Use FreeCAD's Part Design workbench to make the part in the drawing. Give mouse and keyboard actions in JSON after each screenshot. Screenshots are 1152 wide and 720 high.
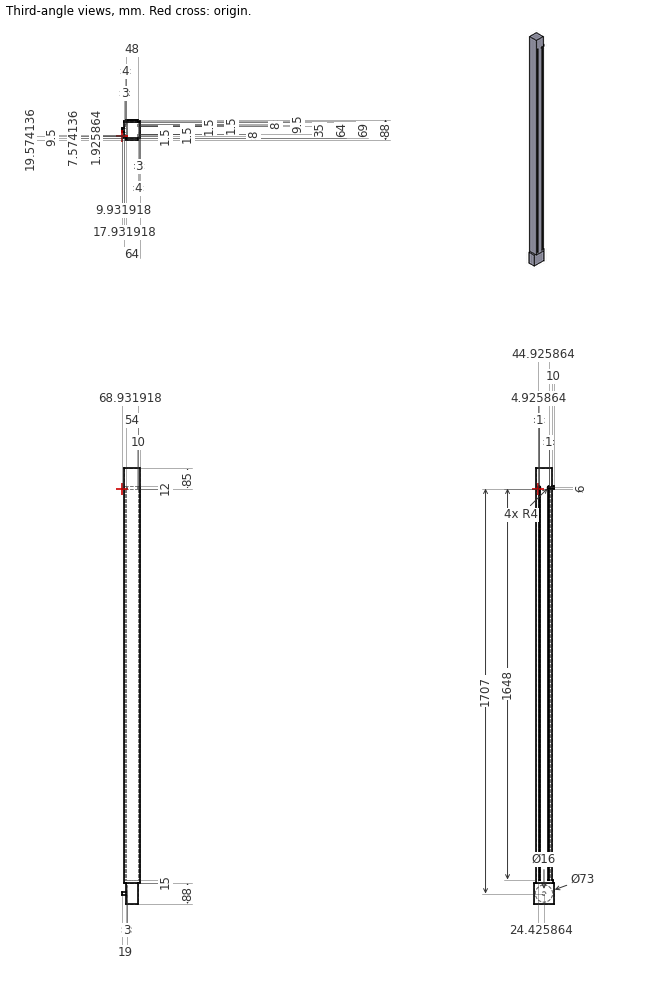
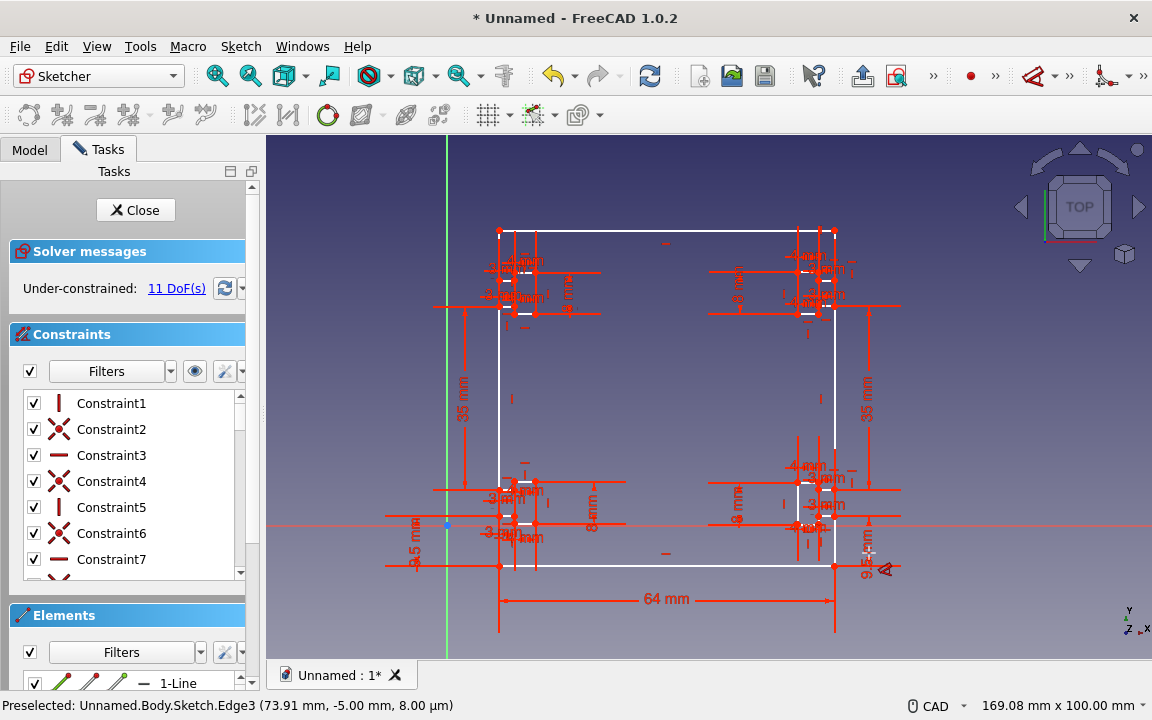
{"action": "scroll", "coordinate": [819, 520], "scroll_direction": "up", "scroll_amount": 9}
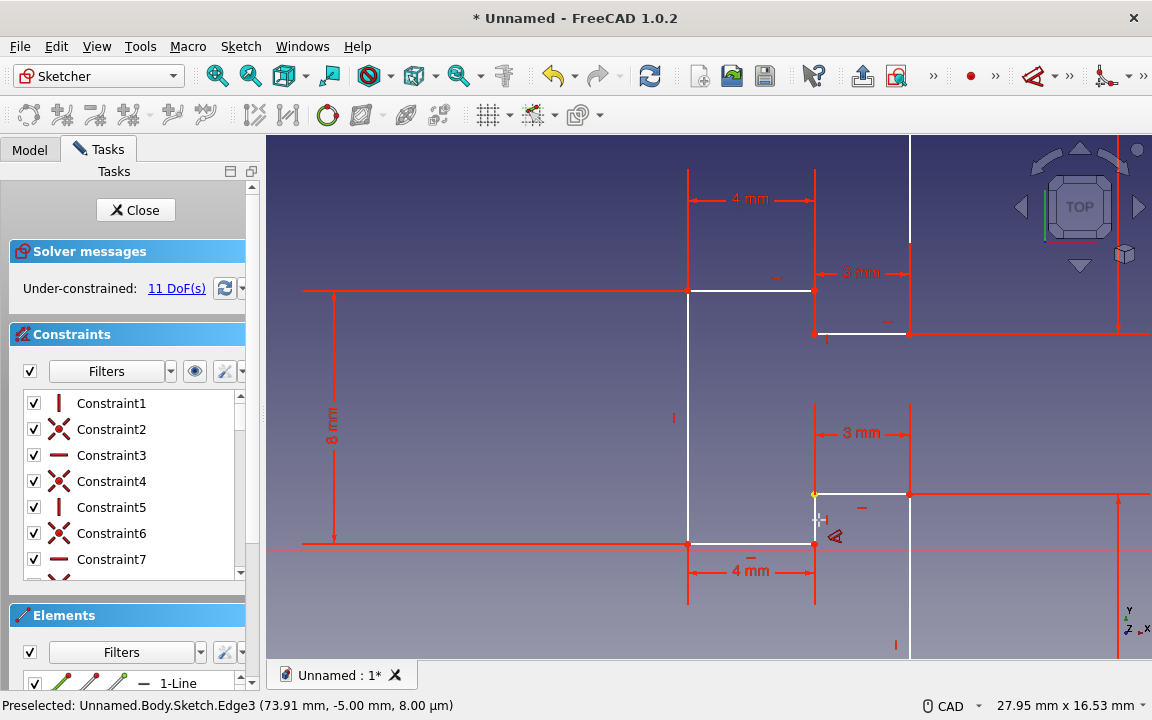
{"action": "left_click", "coordinate": [815, 519]}
{"action": "left_click", "coordinate": [849, 519]}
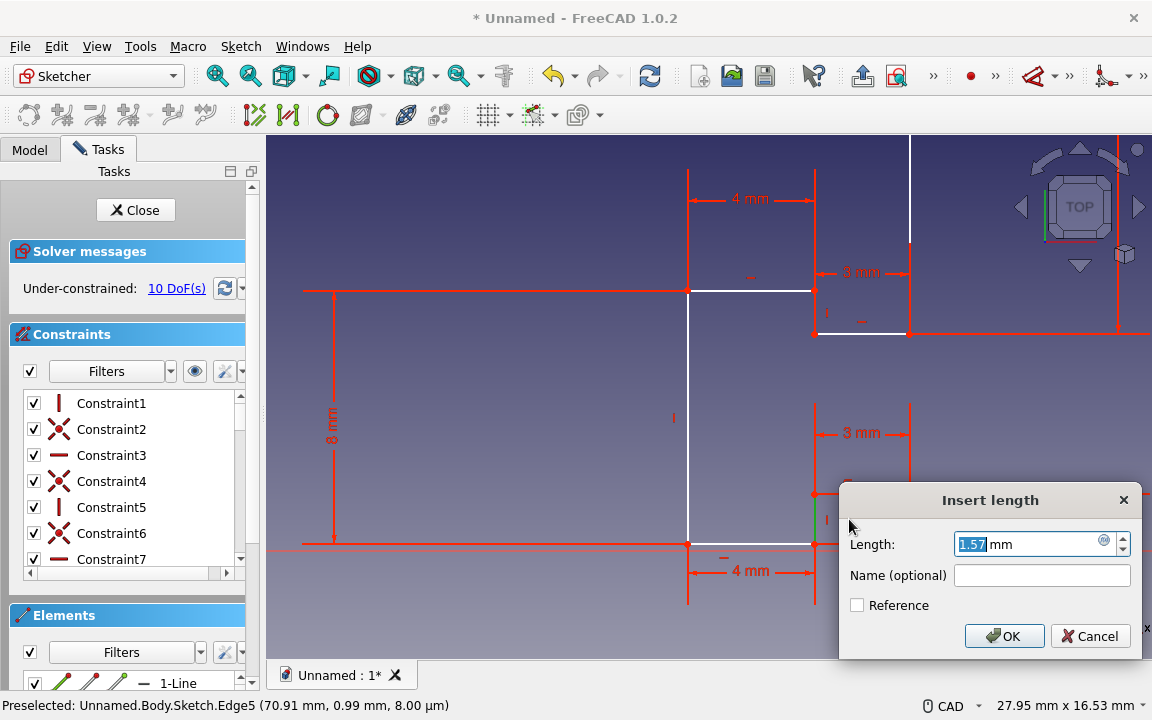
{"action": "type", "text": "1.5"}
{"action": "key", "text": "Return"}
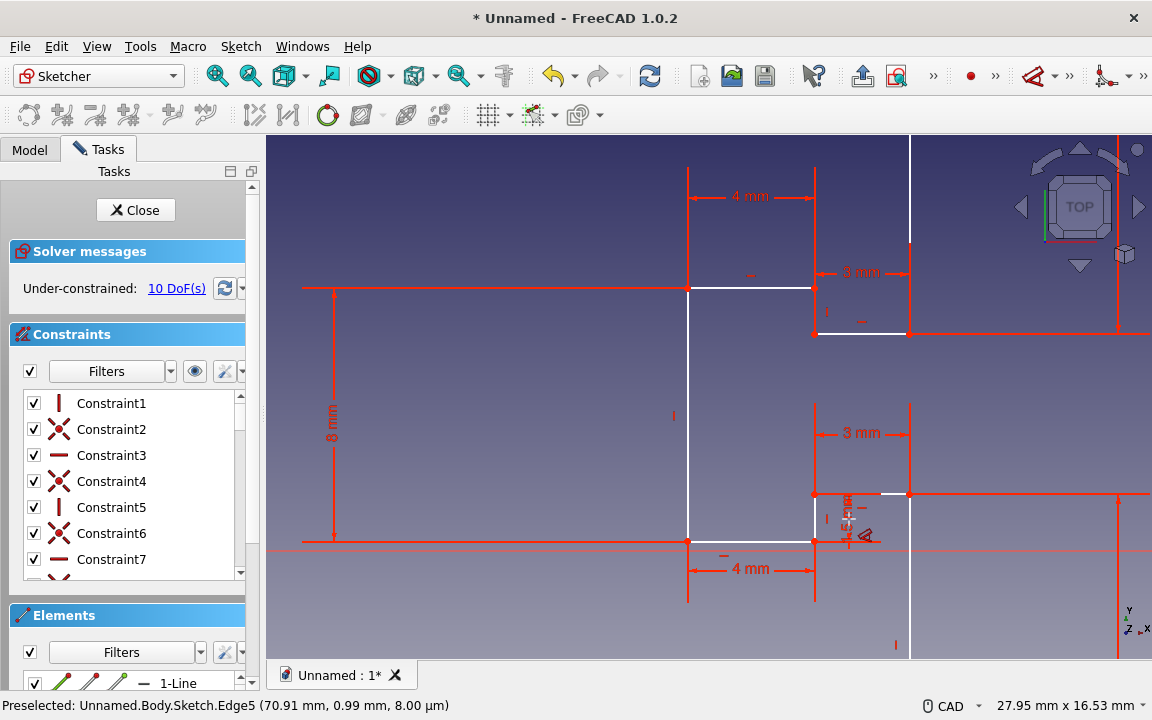
{"action": "left_click", "coordinate": [815, 302]}
{"action": "left_click", "coordinate": [849, 311]}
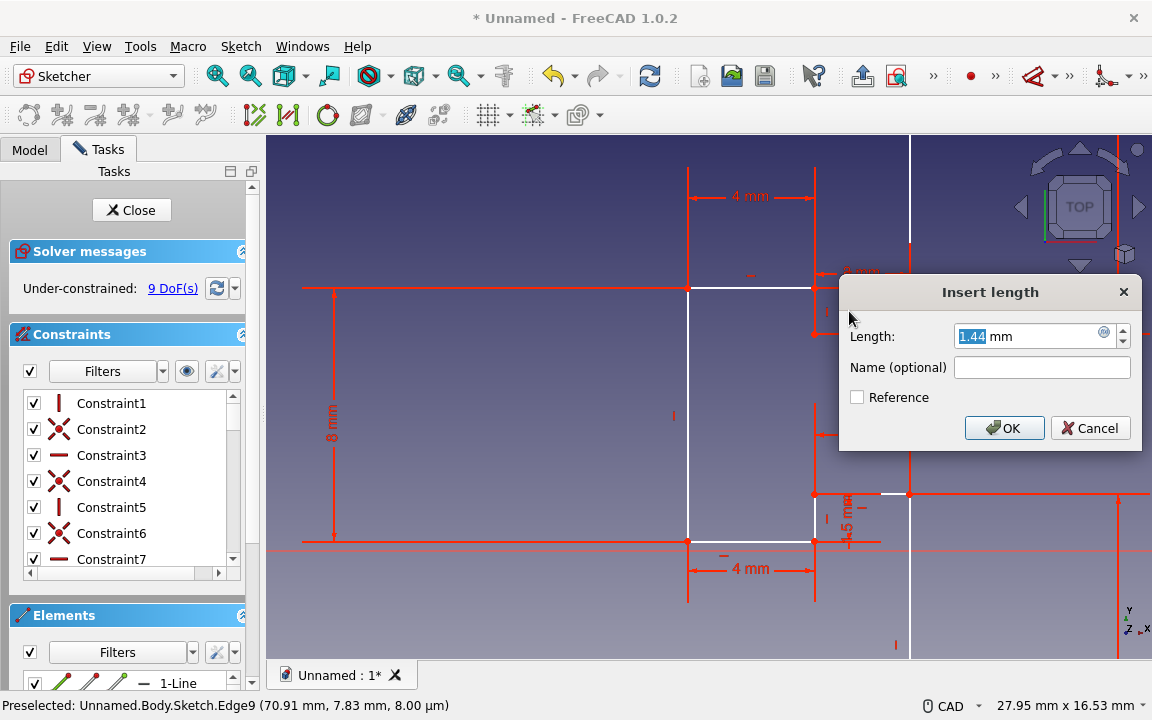
{"action": "type", "text": "1.5"}
{"action": "key", "text": "Return"}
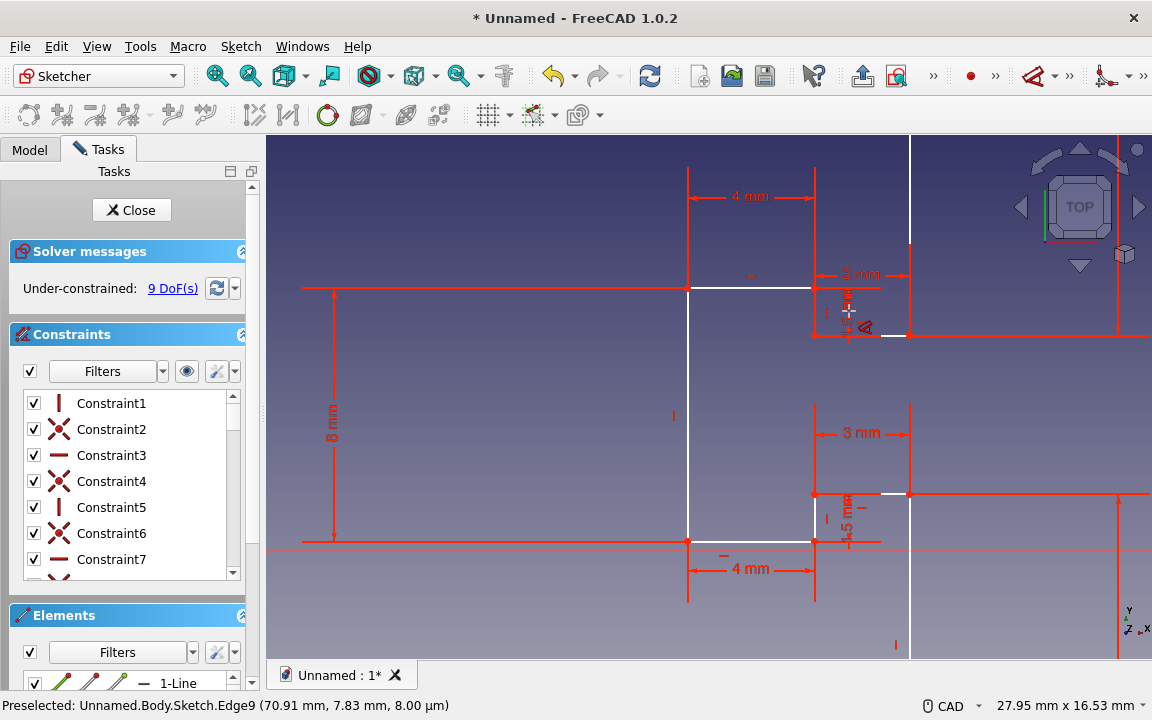
{"action": "scroll", "coordinate": [819, 520], "scroll_direction": "down", "scroll_amount": 9}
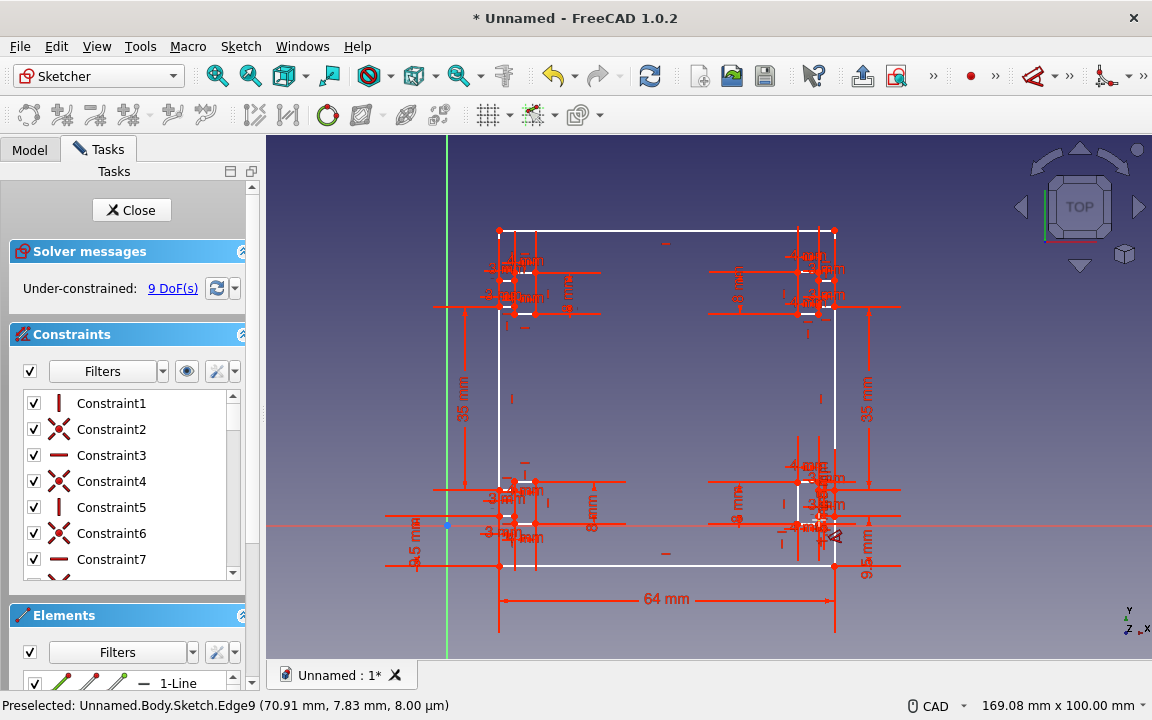
{"action": "scroll", "coordinate": [819, 309], "scroll_direction": "up", "scroll_amount": 10}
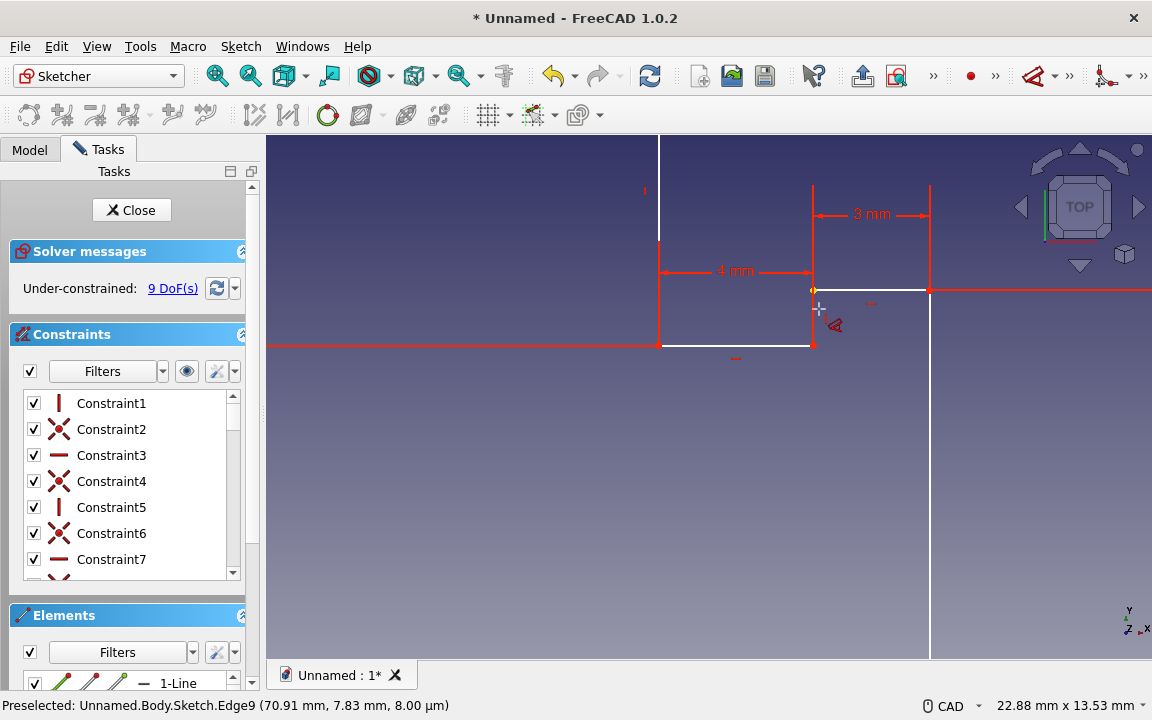
{"action": "left_click", "coordinate": [813, 307]}
{"action": "left_click", "coordinate": [847, 318]}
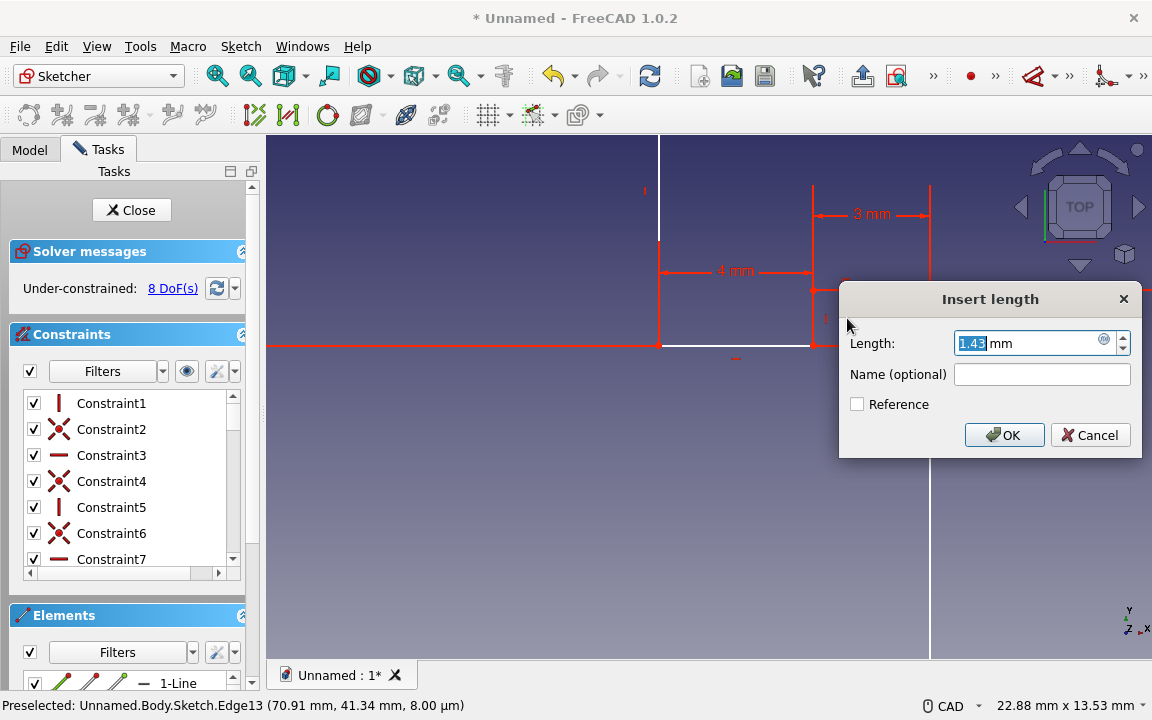
{"action": "type", "text": "1.5"}
{"action": "key", "text": "Return"}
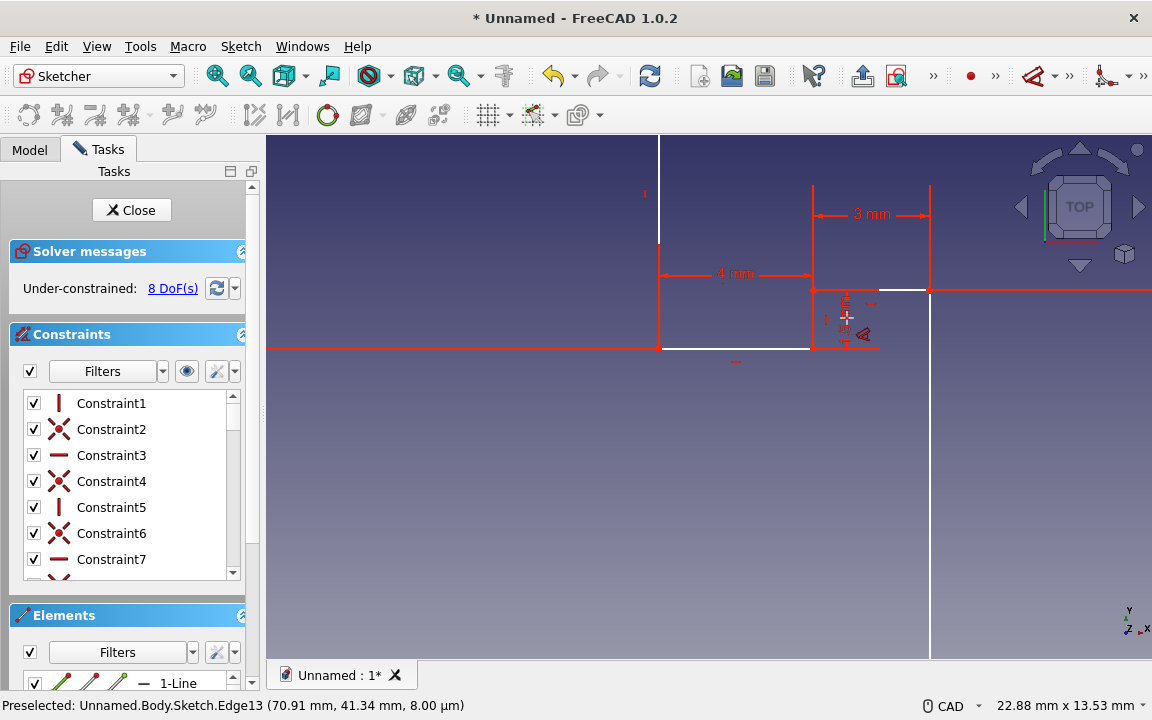
{"action": "scroll", "coordinate": [819, 308], "scroll_direction": "down", "scroll_amount": 10}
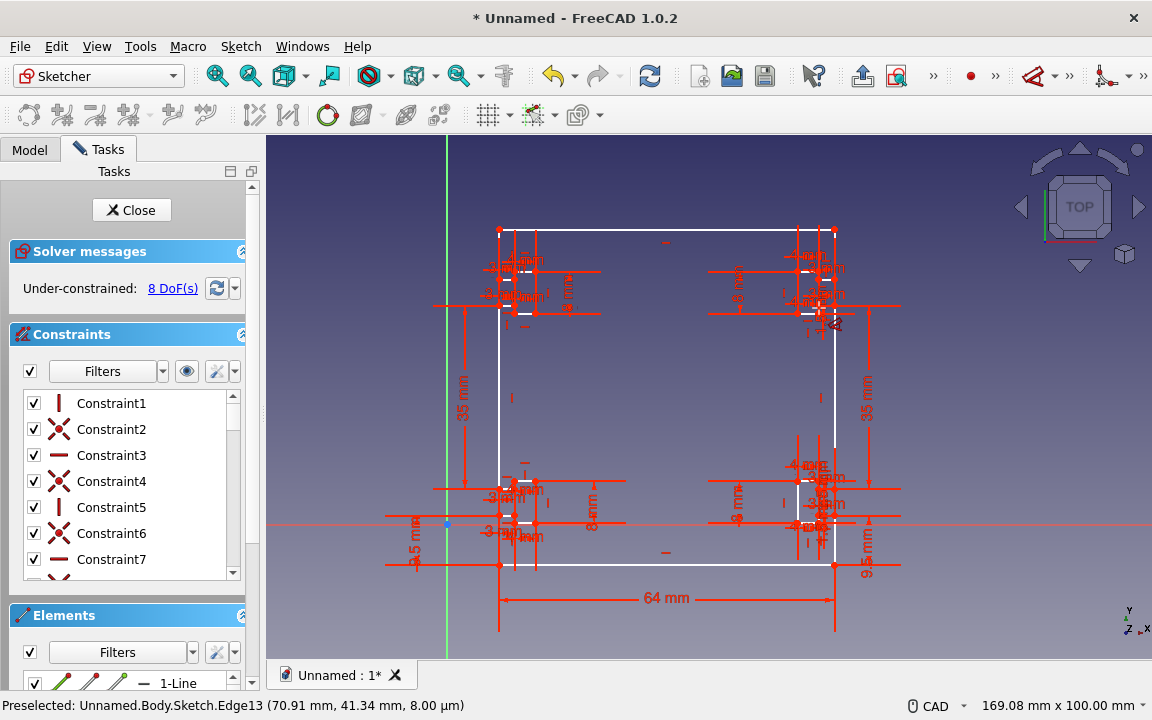
{"action": "scroll", "coordinate": [819, 274], "scroll_direction": "up", "scroll_amount": 9}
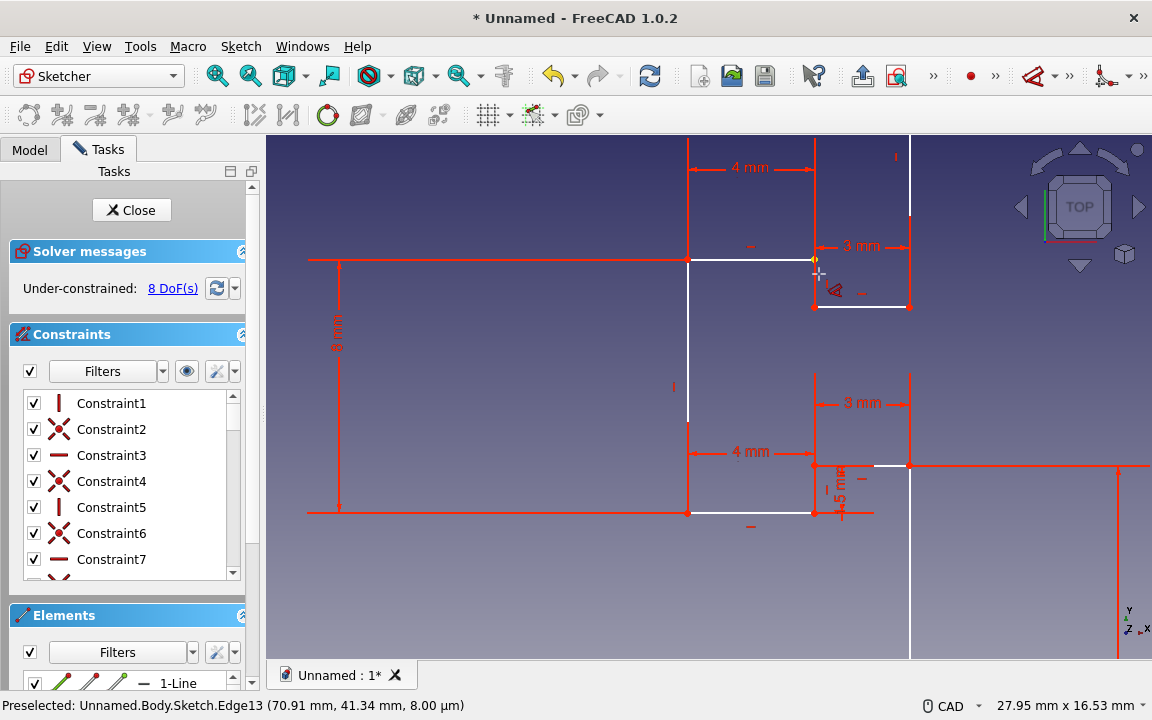
{"action": "left_click", "coordinate": [815, 274]}
{"action": "left_click", "coordinate": [849, 283]}